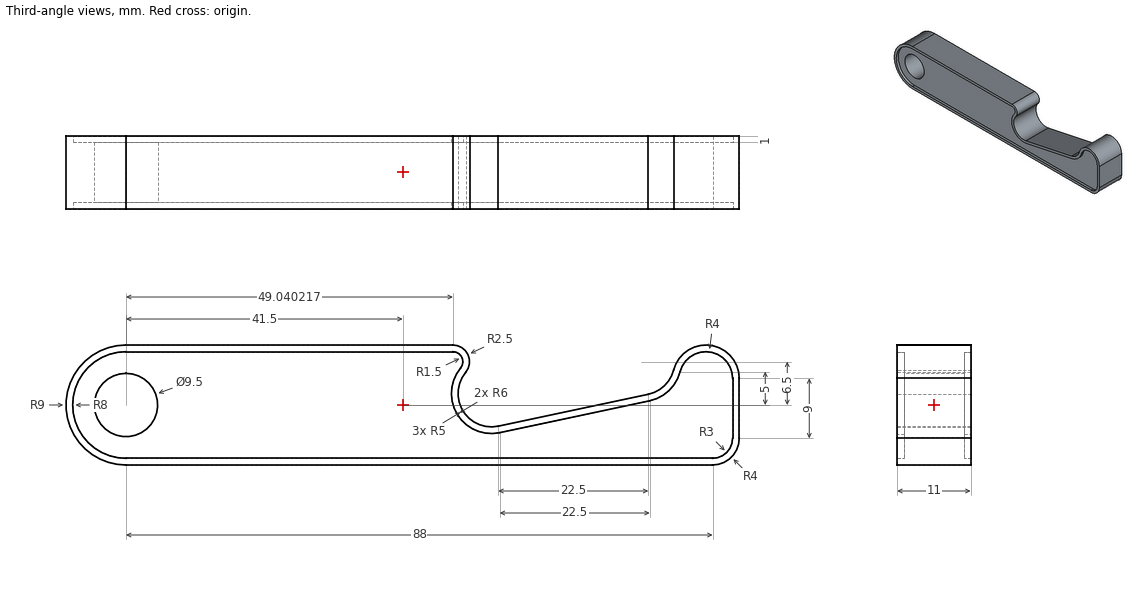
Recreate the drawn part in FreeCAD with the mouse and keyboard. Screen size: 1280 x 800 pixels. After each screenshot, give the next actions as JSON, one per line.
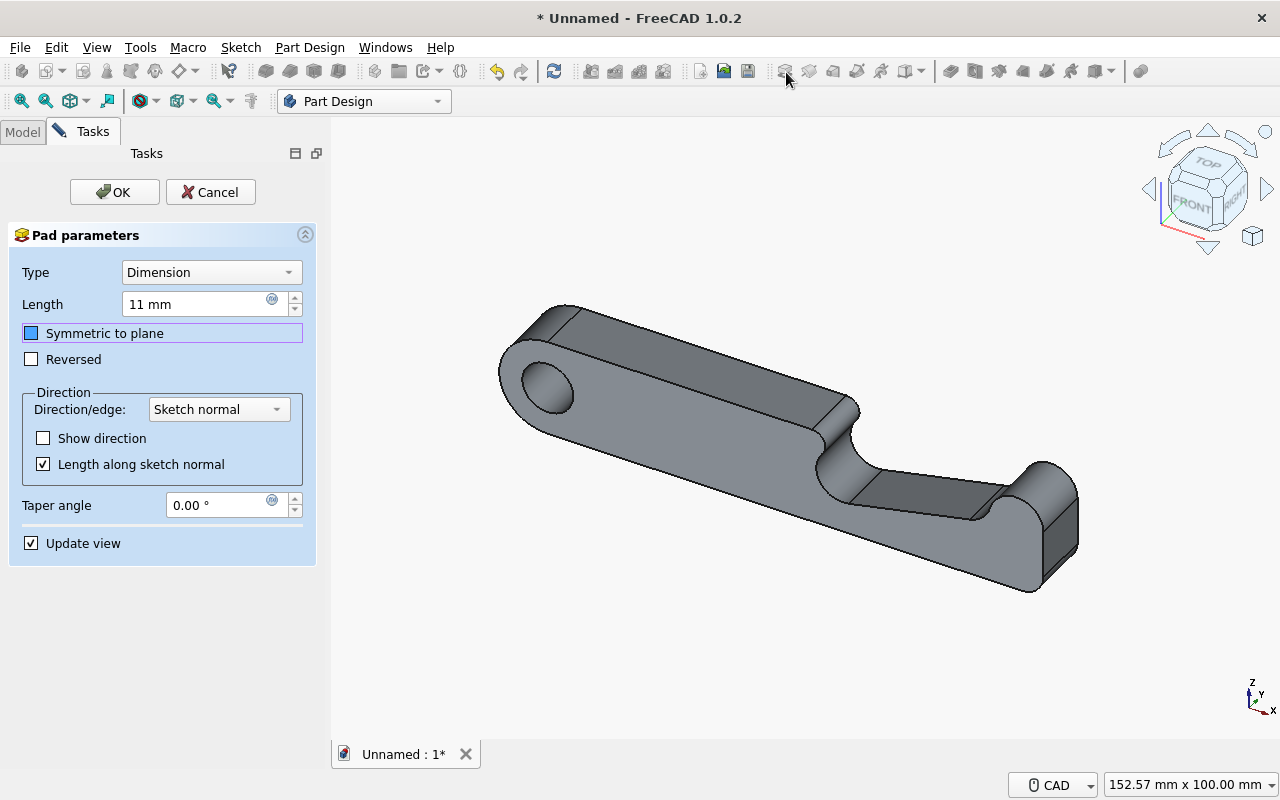
{"action": "left_click", "coordinate": [30, 333]}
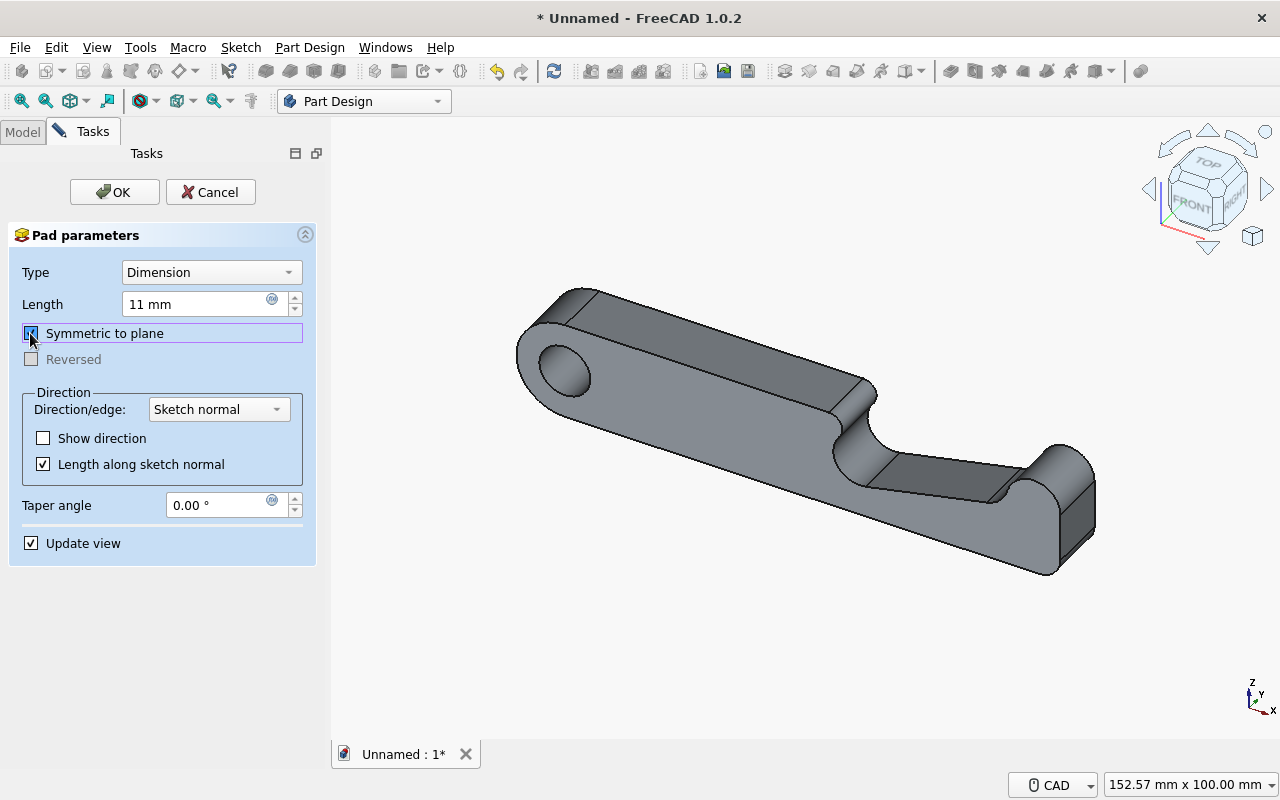
{"action": "left_click", "coordinate": [115, 192]}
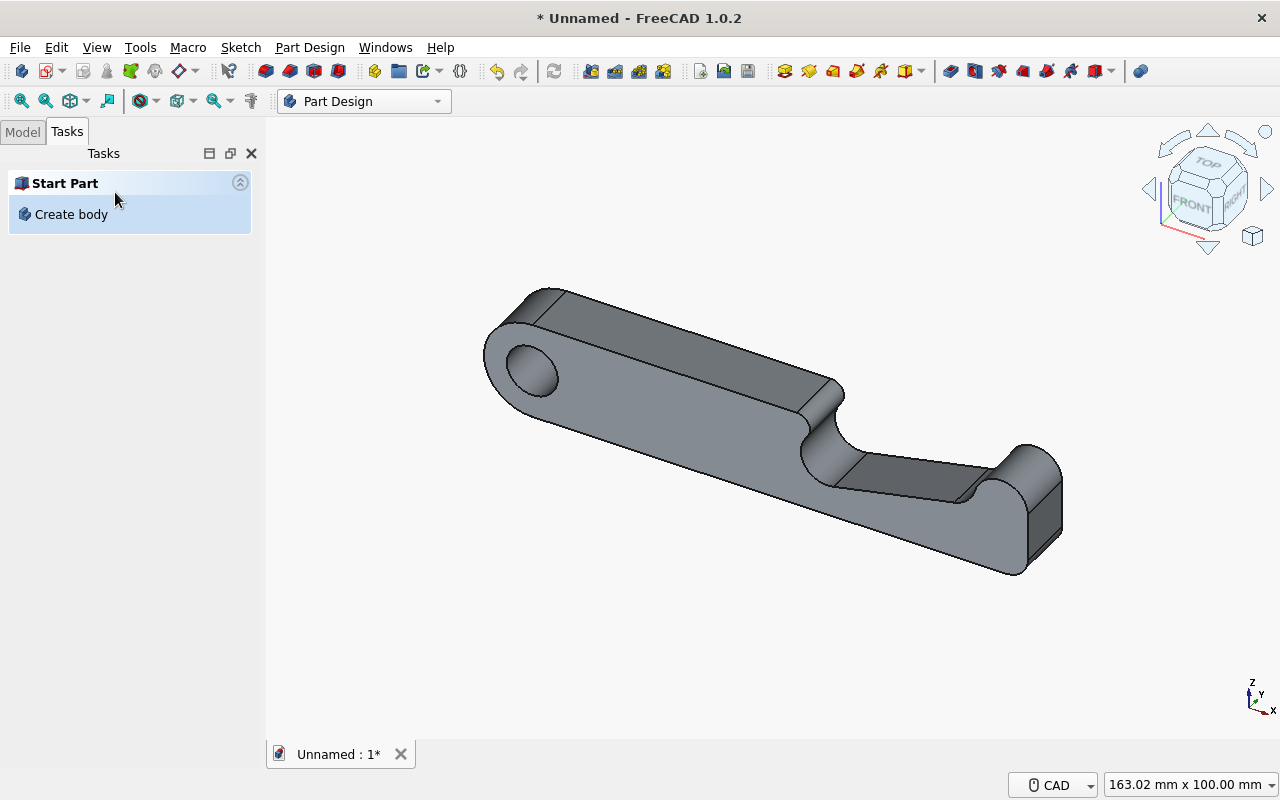
{"action": "key", "text": "4"}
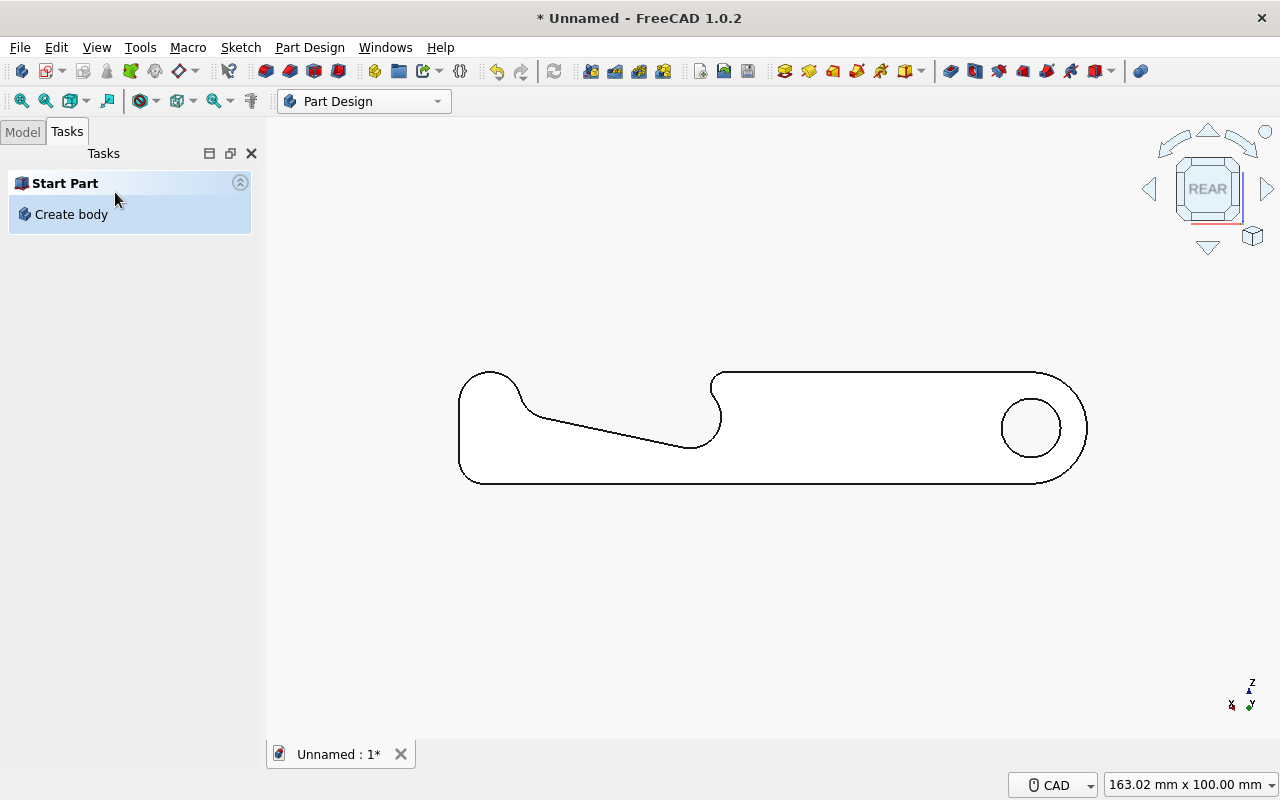
{"action": "left_click", "coordinate": [863, 427]}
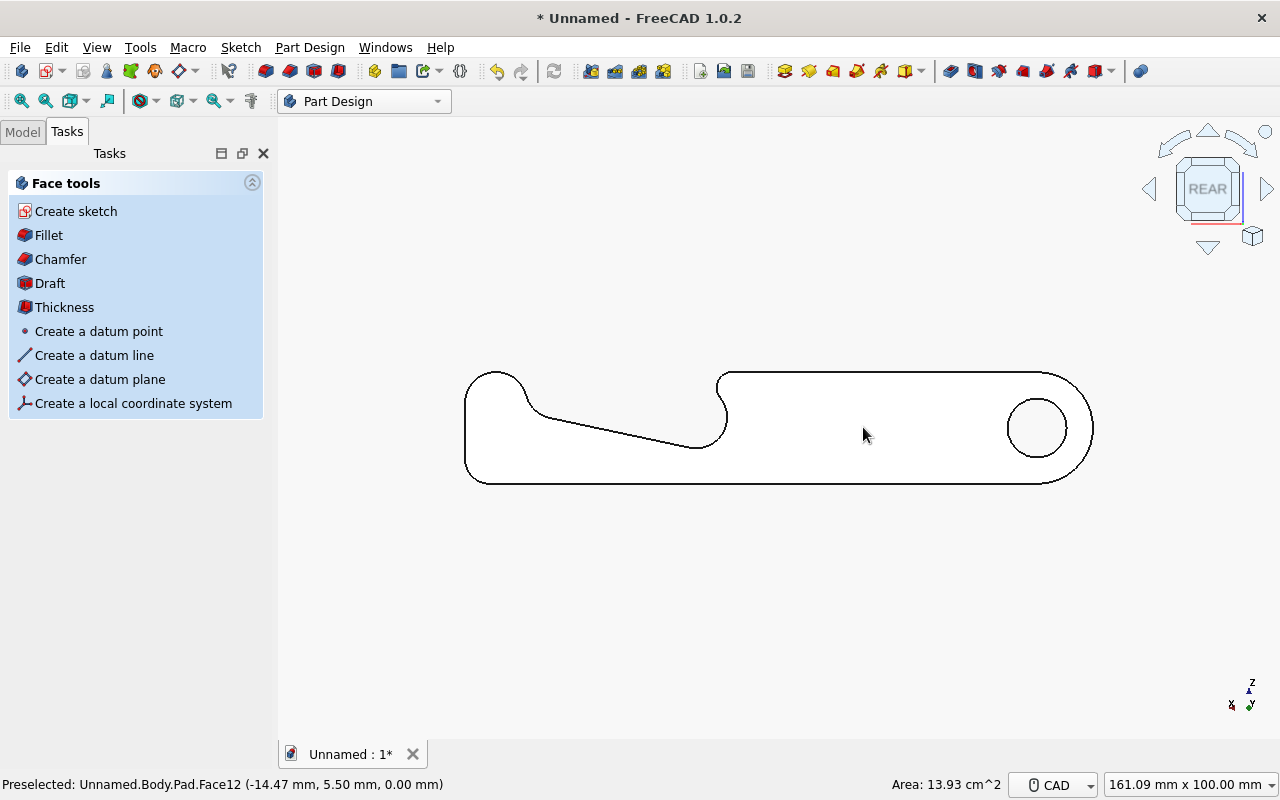
{"action": "left_click", "coordinate": [46, 72]}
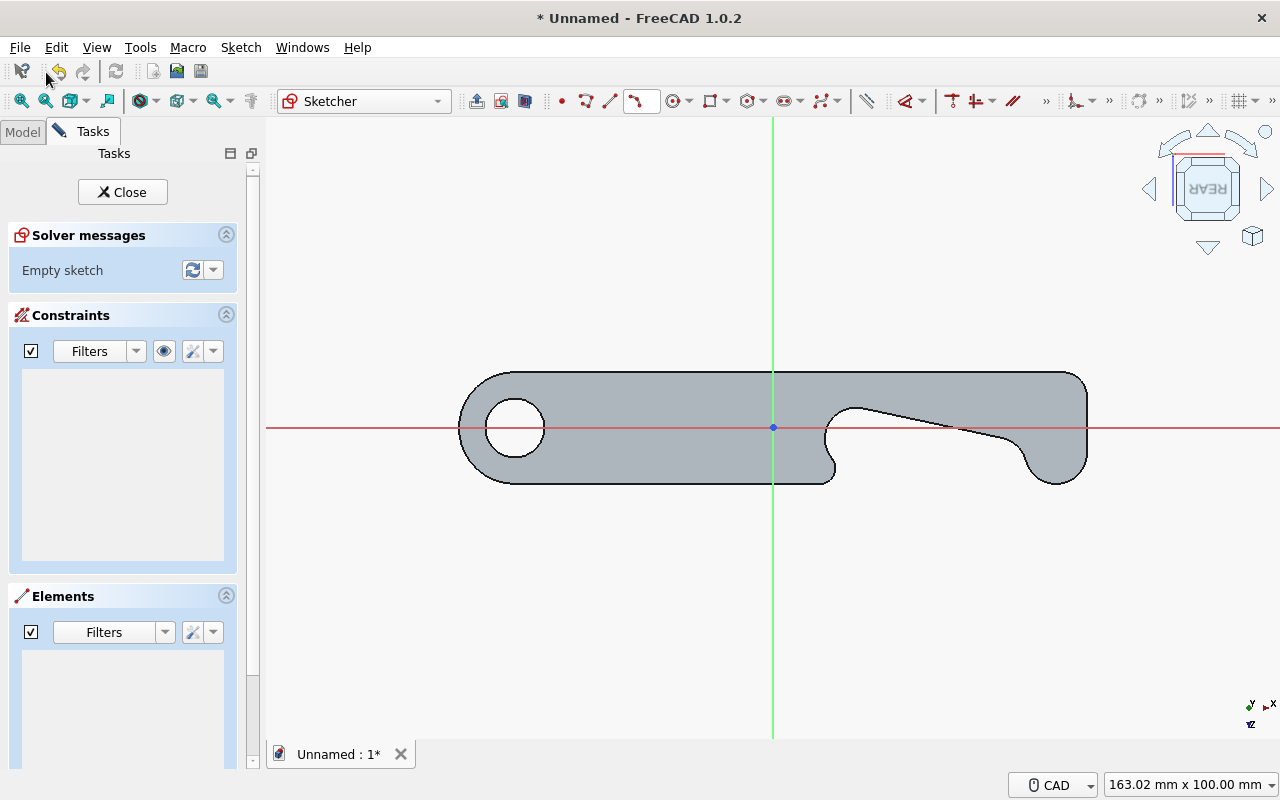
{"action": "left_click", "coordinate": [610, 102]}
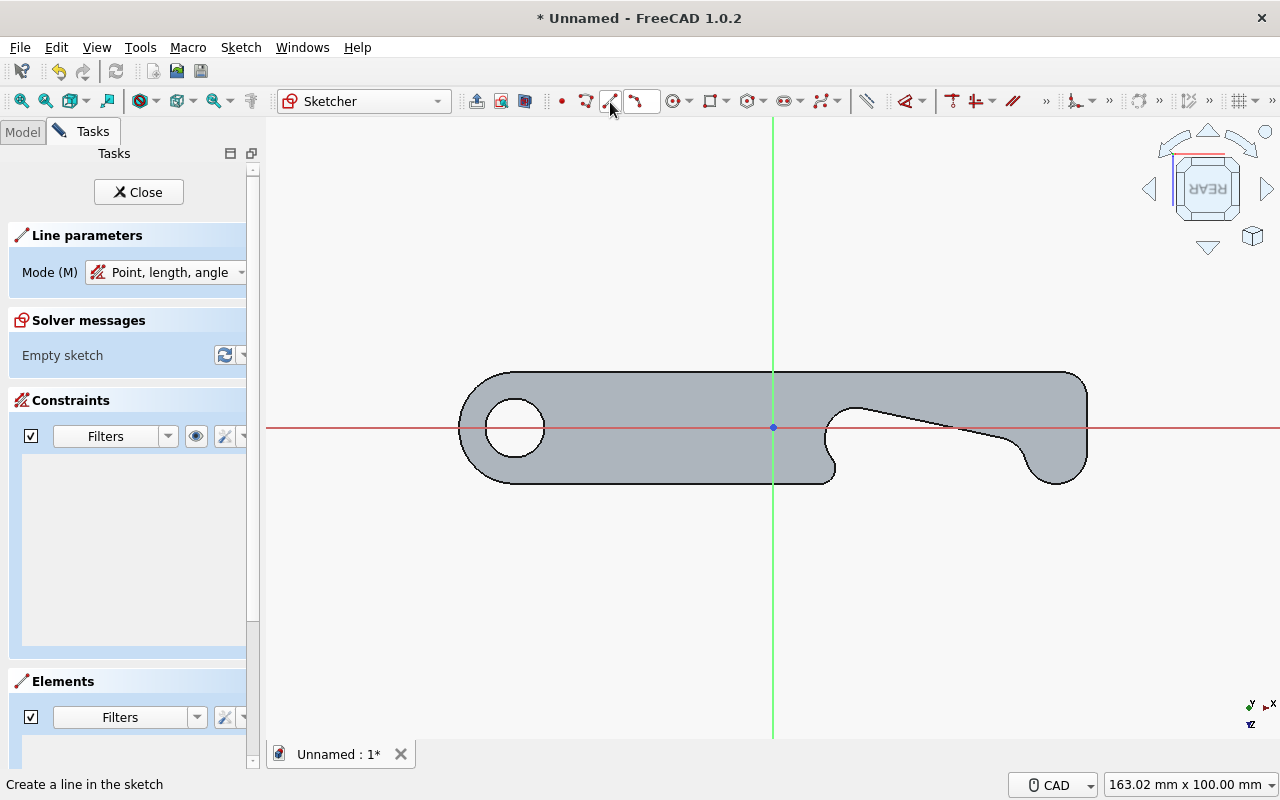
{"action": "left_click", "coordinate": [515, 478]}
{"action": "left_click", "coordinate": [820, 478]}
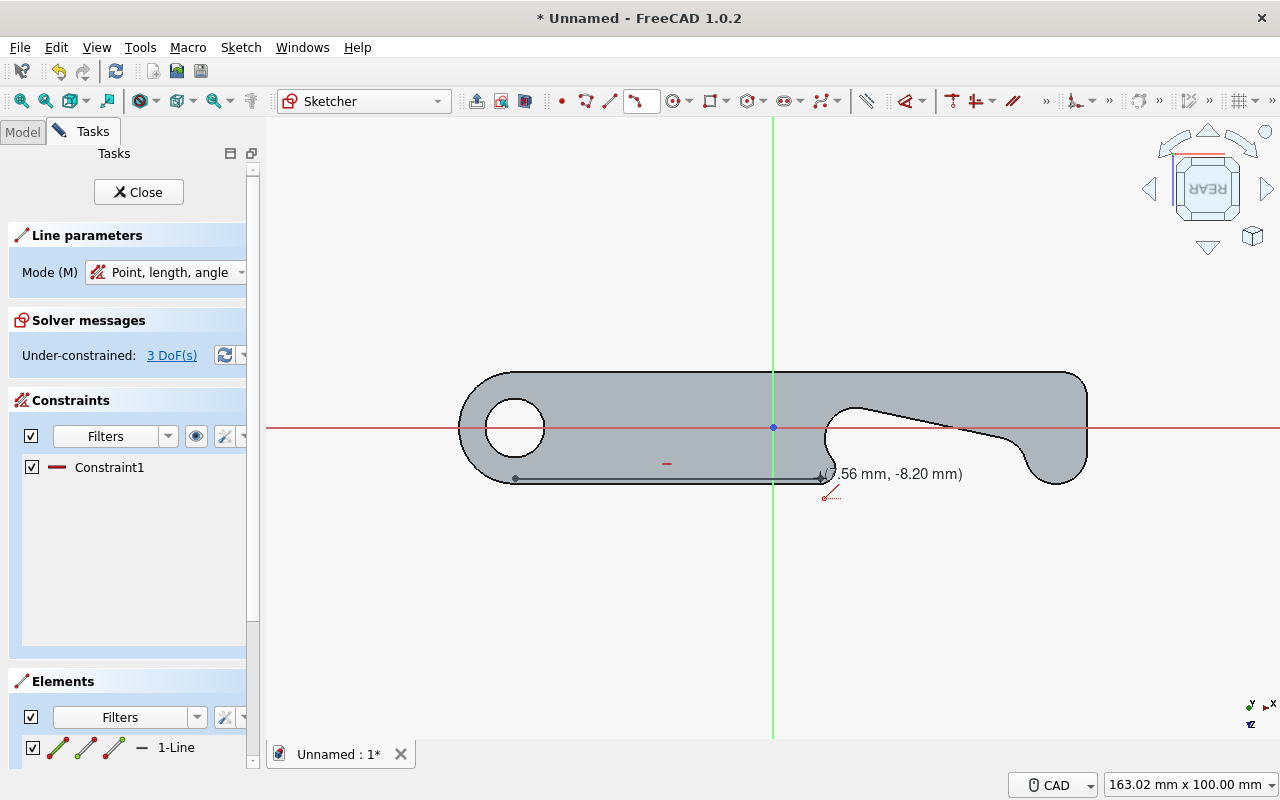
{"action": "left_click", "coordinate": [864, 402]}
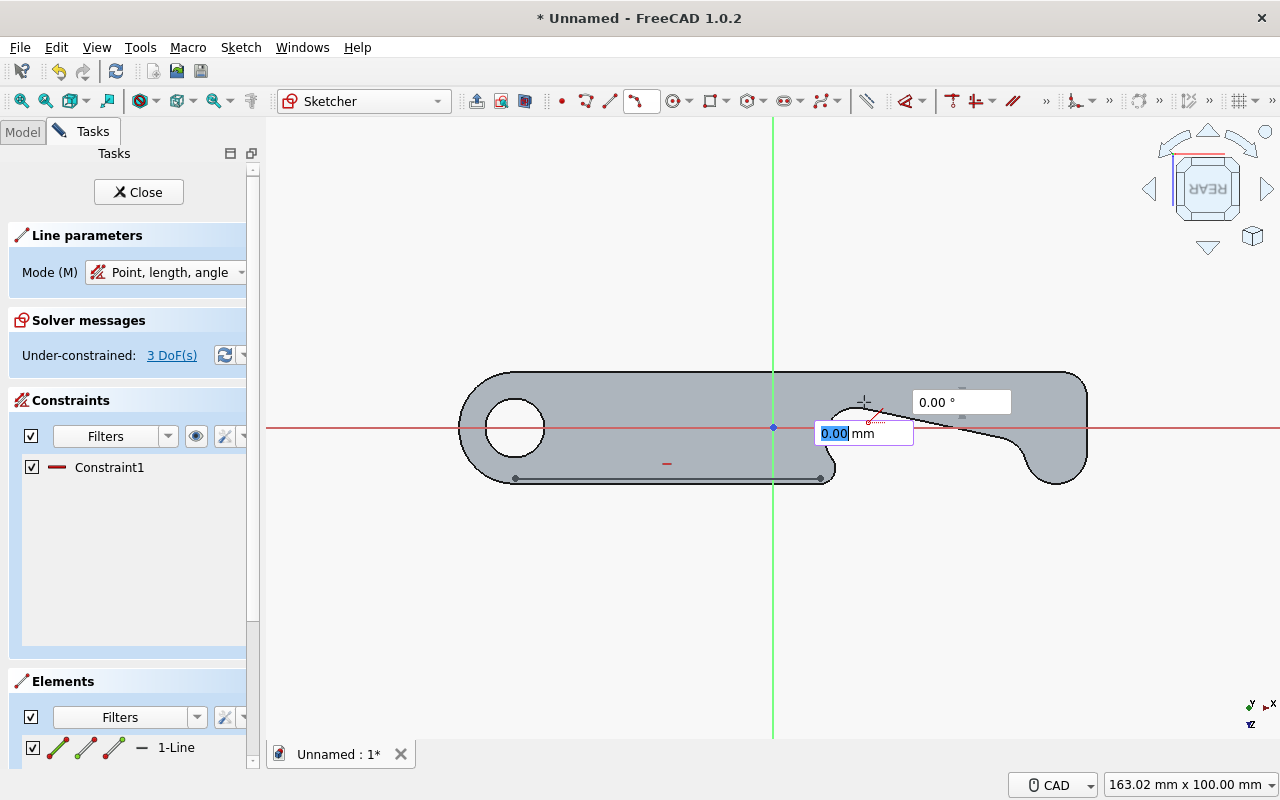
{"action": "scroll", "coordinate": [1004, 432], "scroll_direction": "up", "scroll_amount": 7}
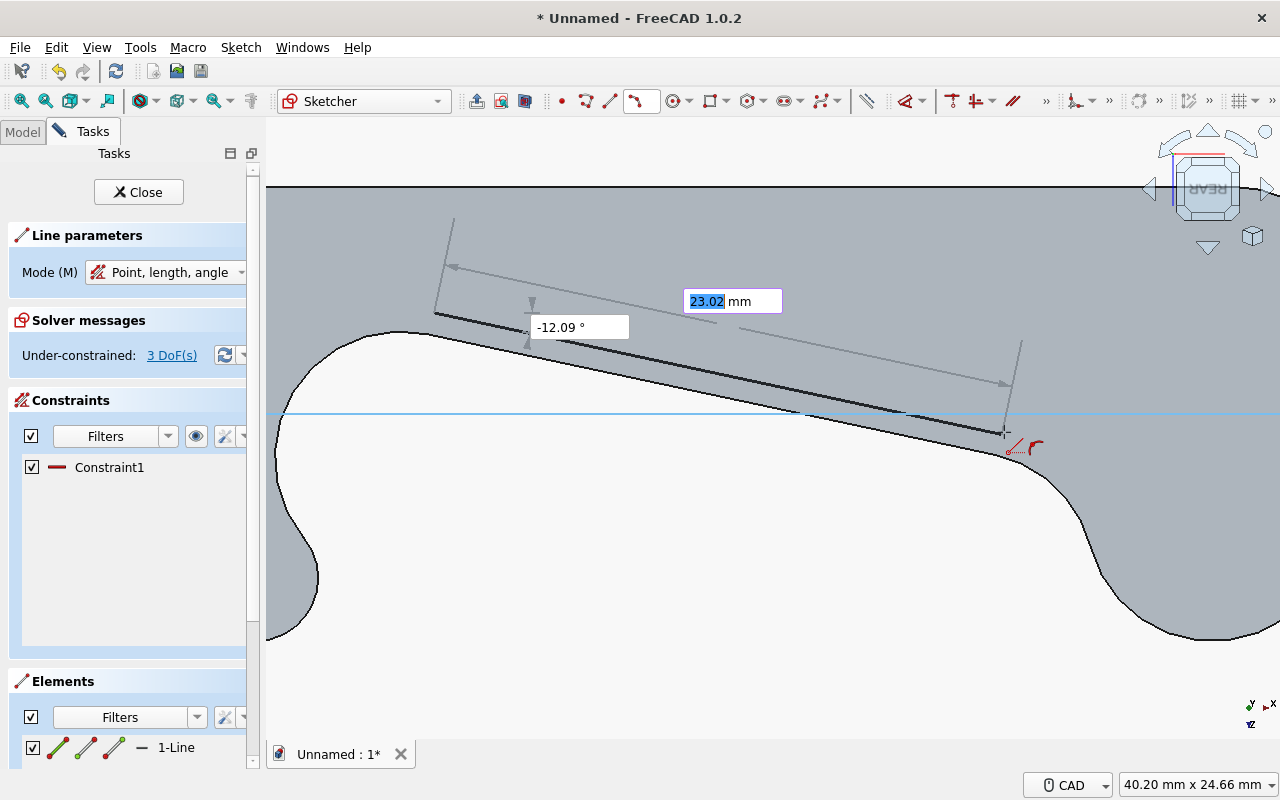
{"action": "left_click", "coordinate": [1000, 430]}